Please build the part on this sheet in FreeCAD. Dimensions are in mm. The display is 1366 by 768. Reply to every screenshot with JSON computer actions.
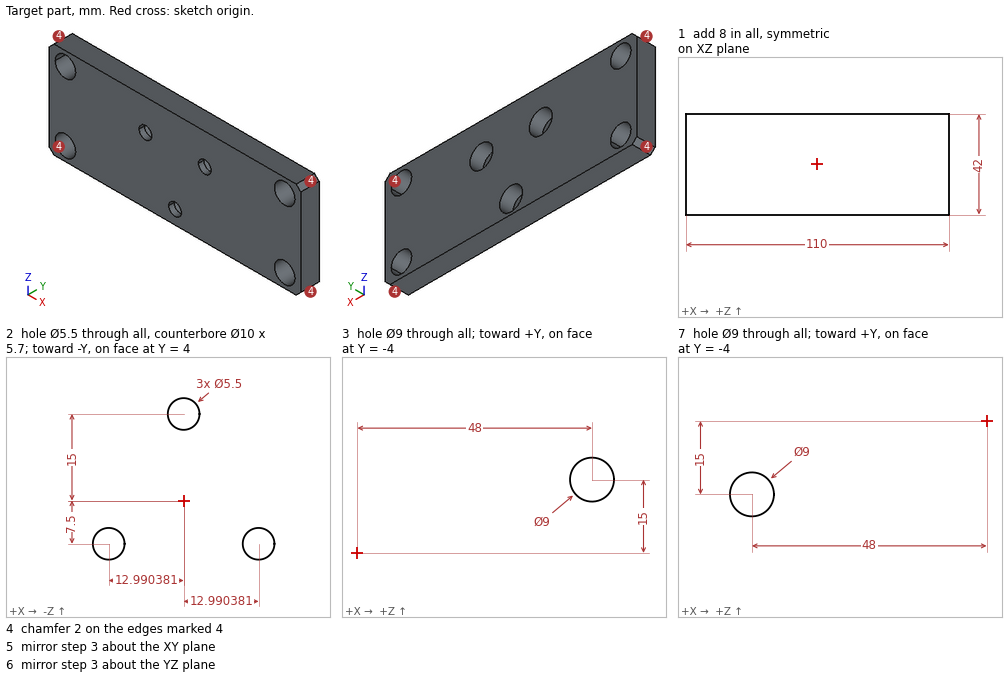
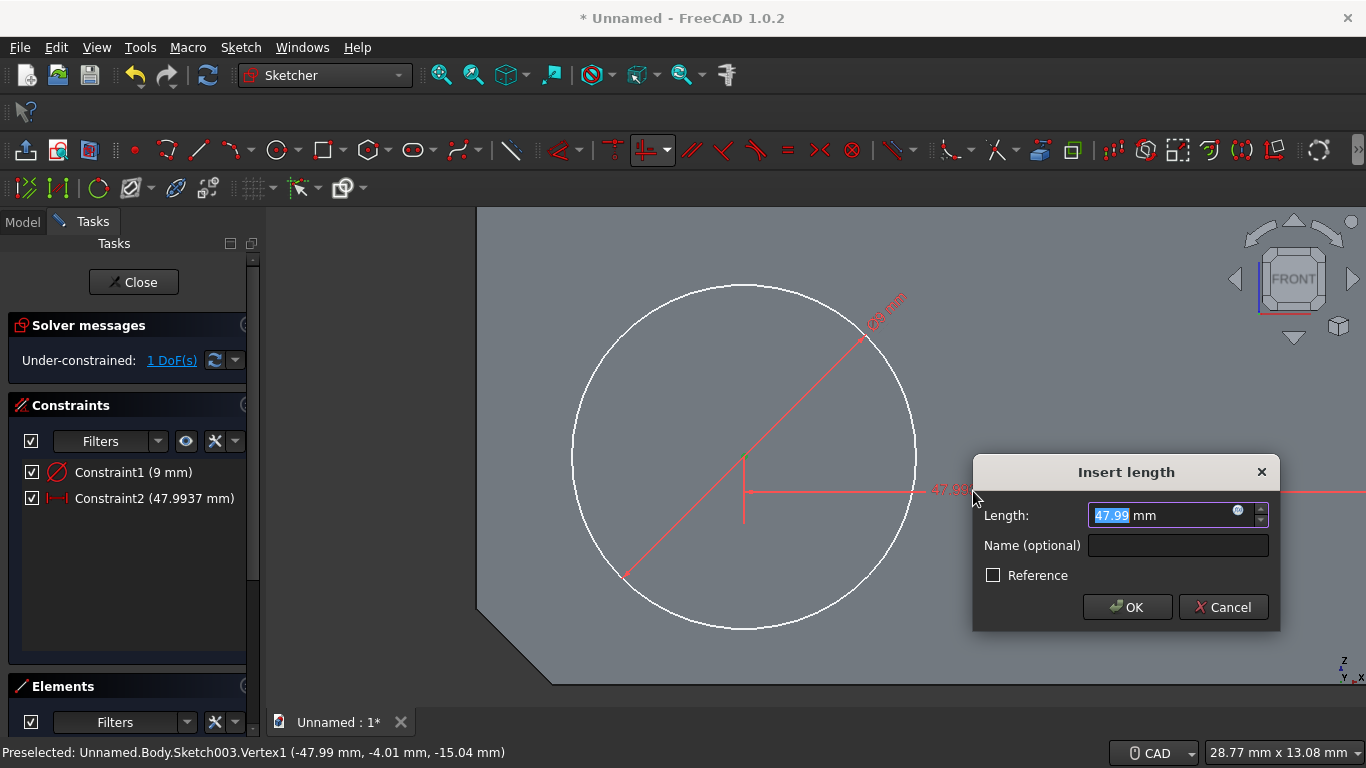
{"action": "type", "text": "48"}
{"action": "key", "text": "Return"}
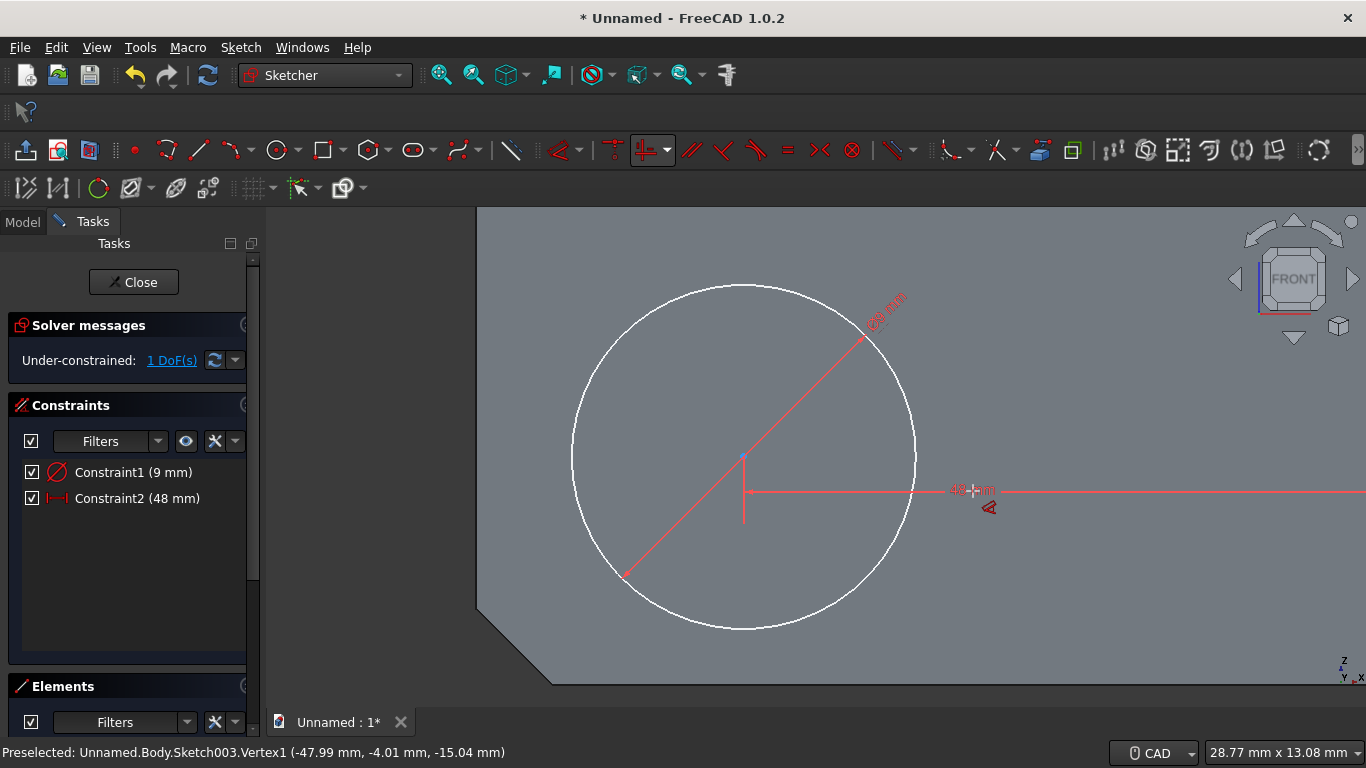
{"action": "left_click", "coordinate": [744, 457]}
{"action": "left_click", "coordinate": [710, 346]}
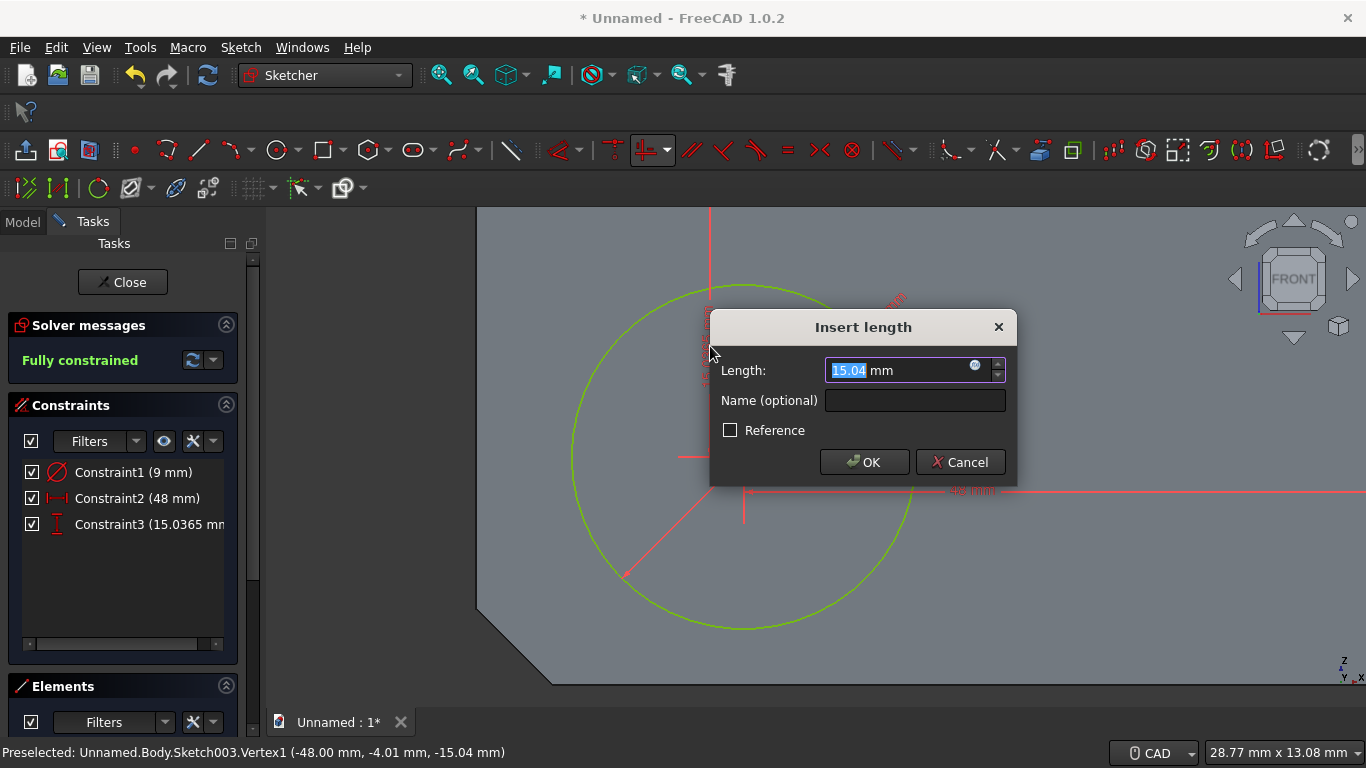
{"action": "type", "text": "15"}
{"action": "key", "text": "Return"}
{"action": "key", "text": "Escape"}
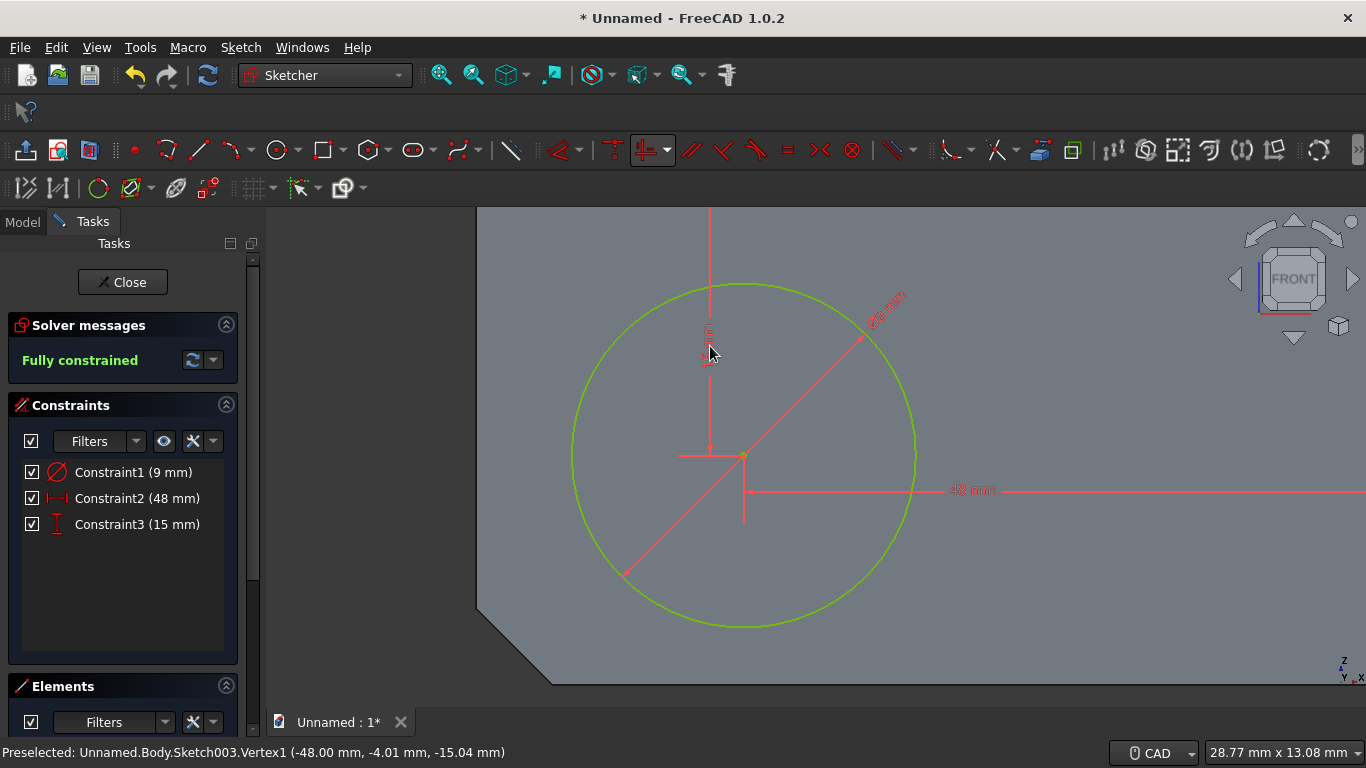
{"action": "left_click", "coordinate": [123, 282]}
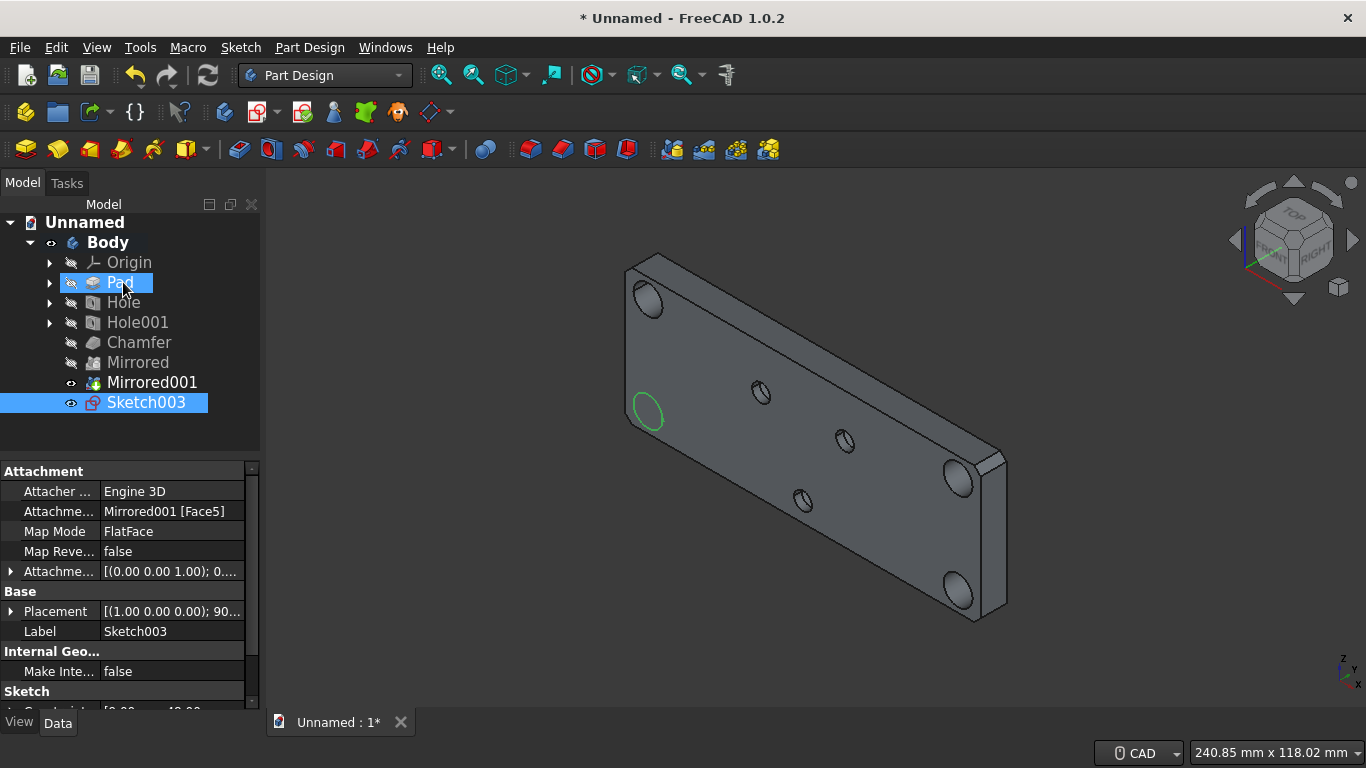
{"action": "left_click", "coordinate": [272, 150]}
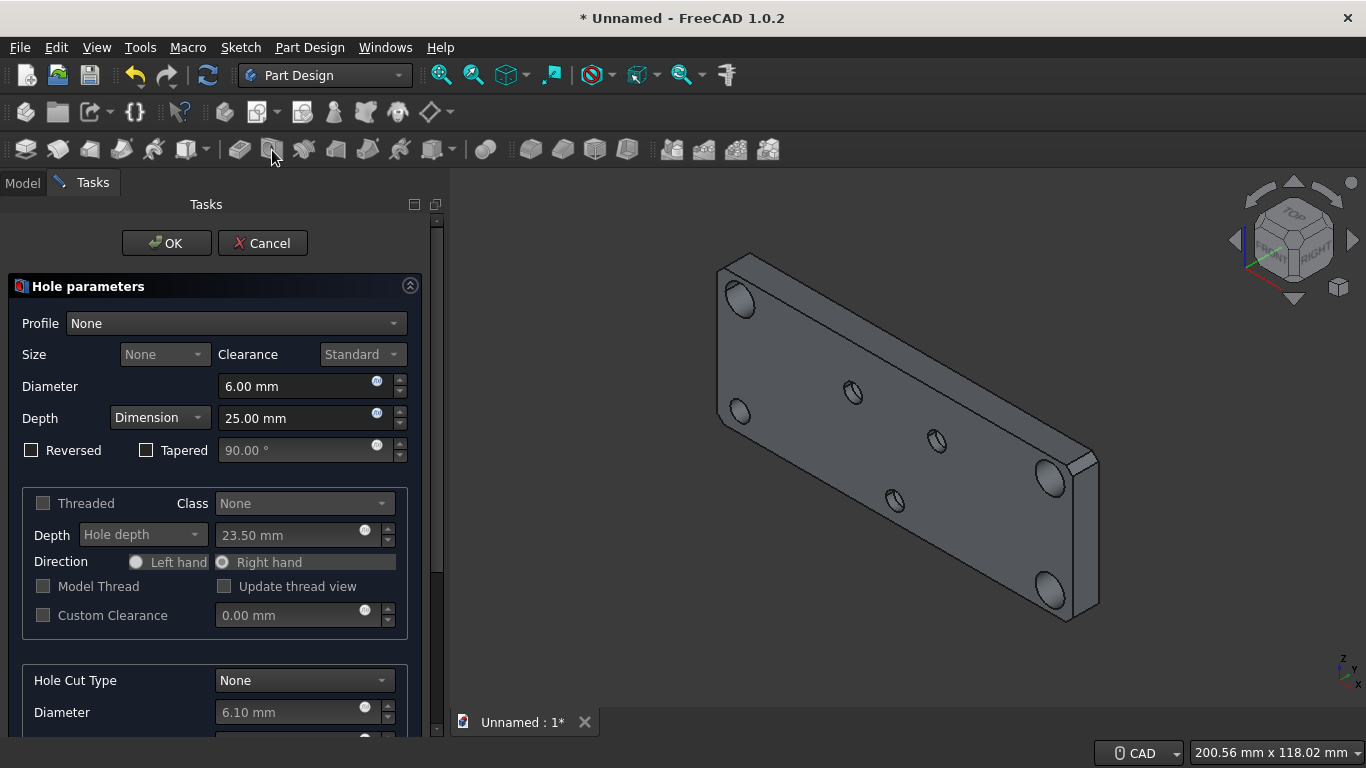
{"action": "triple_click", "coordinate": [305, 386]}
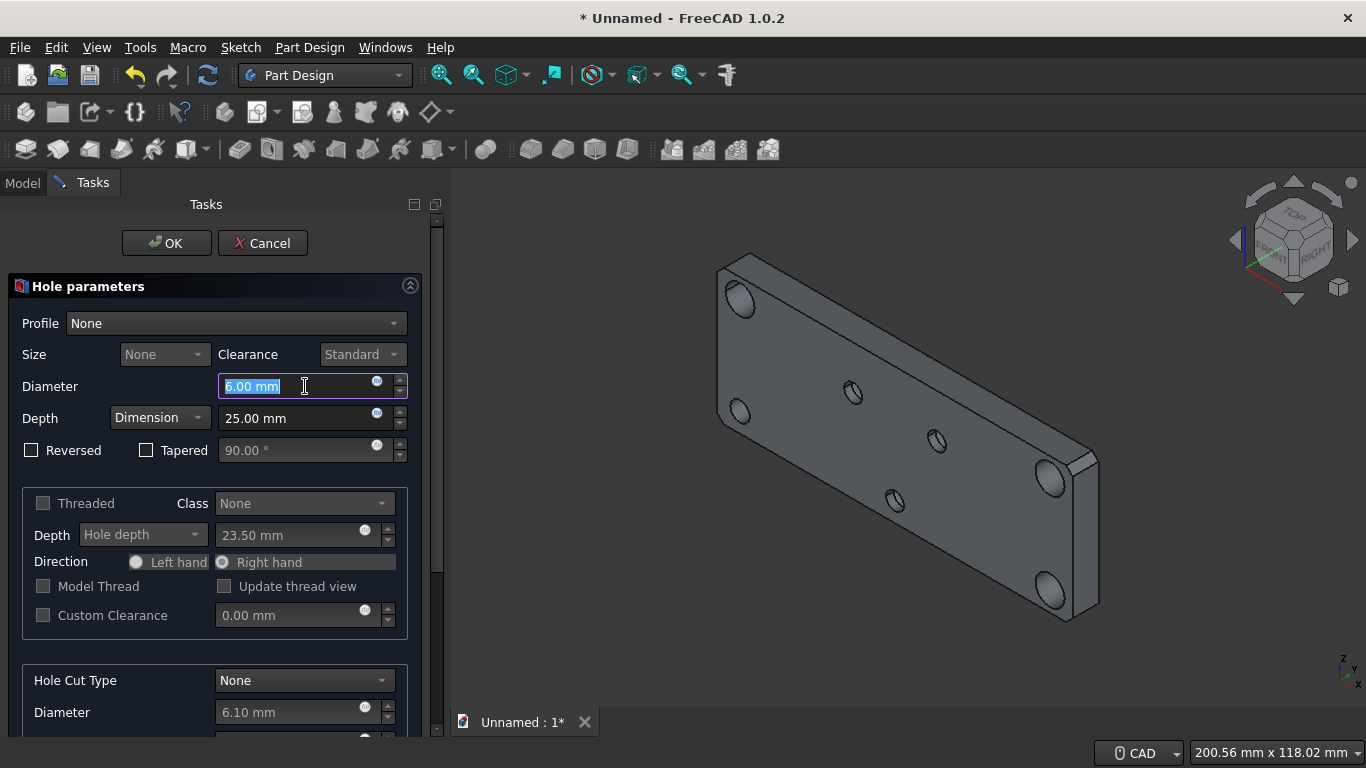
{"action": "type", "text": "9"}
{"action": "key", "text": "Tab"}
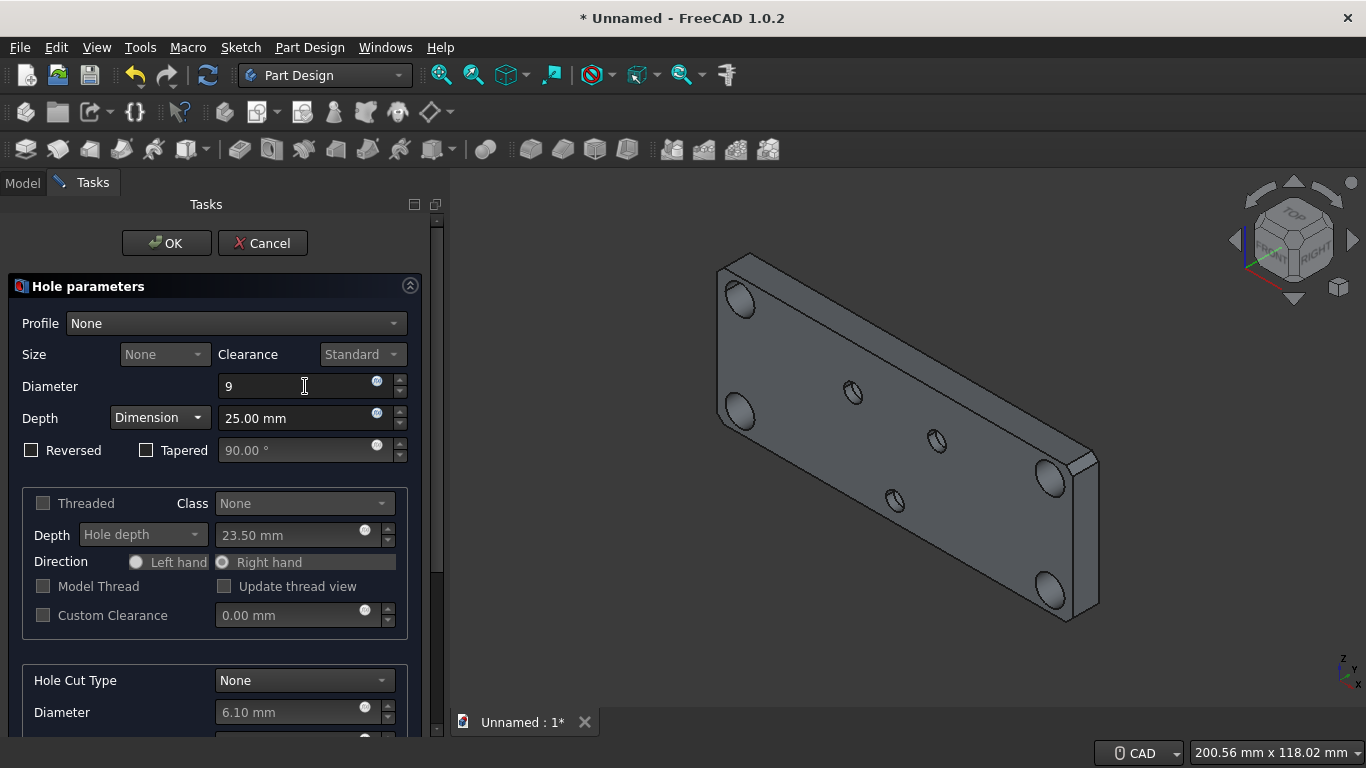
{"action": "left_click", "coordinate": [161, 418]}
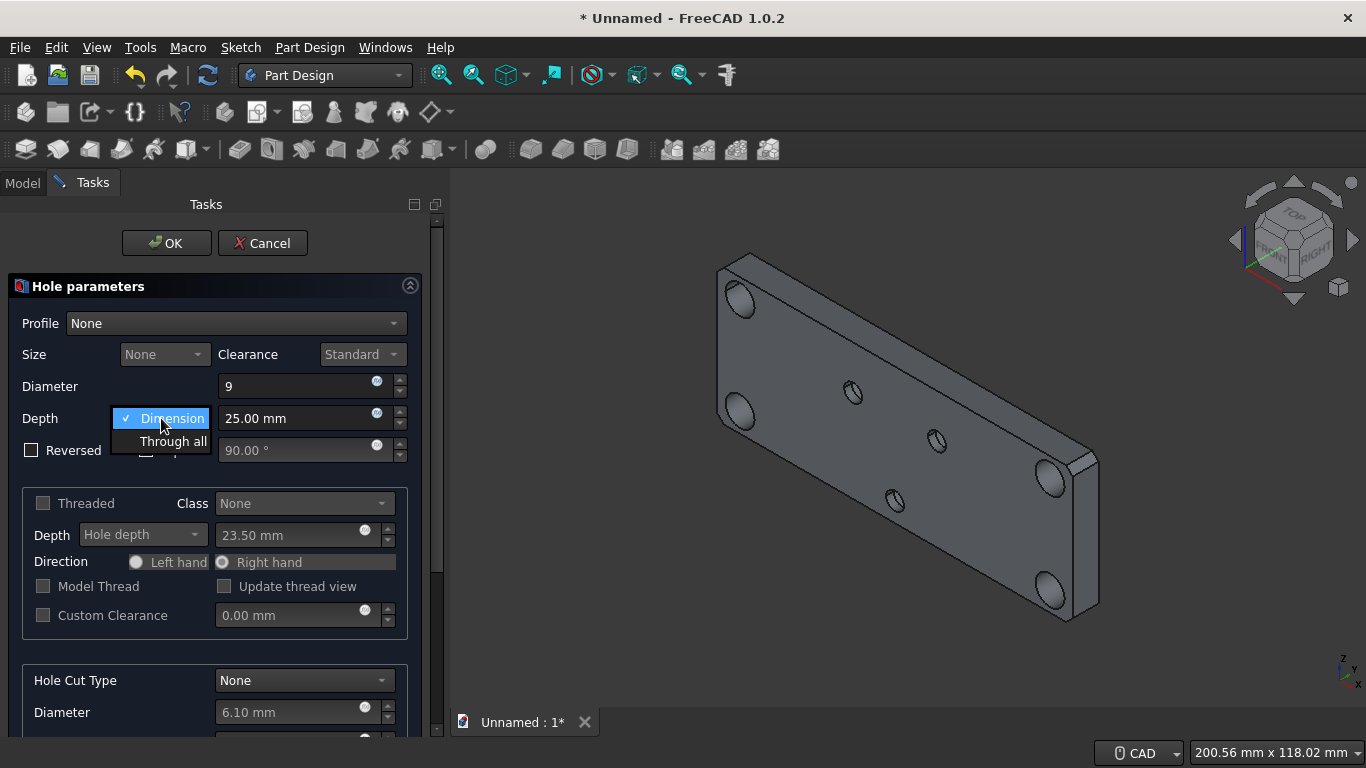
{"action": "left_click", "coordinate": [160, 442]}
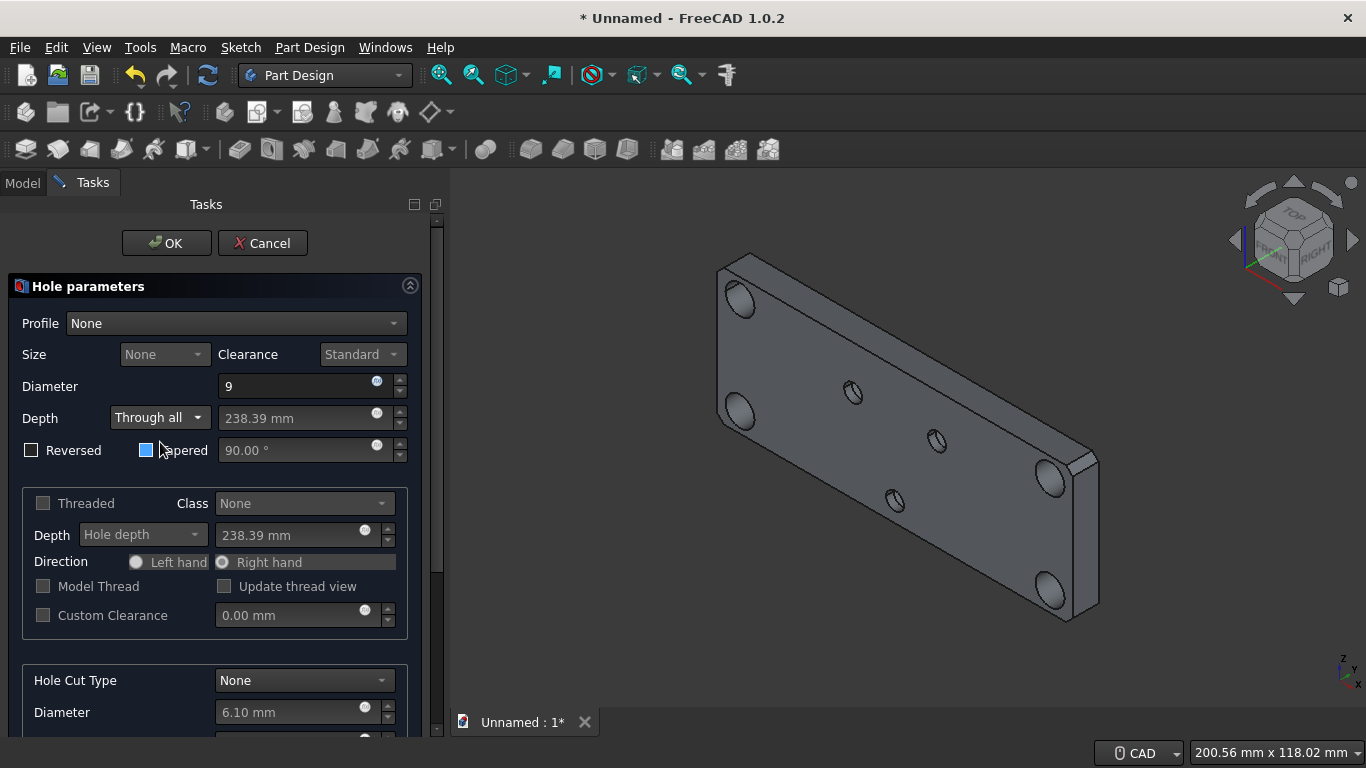
{"action": "left_click", "coordinate": [167, 243]}